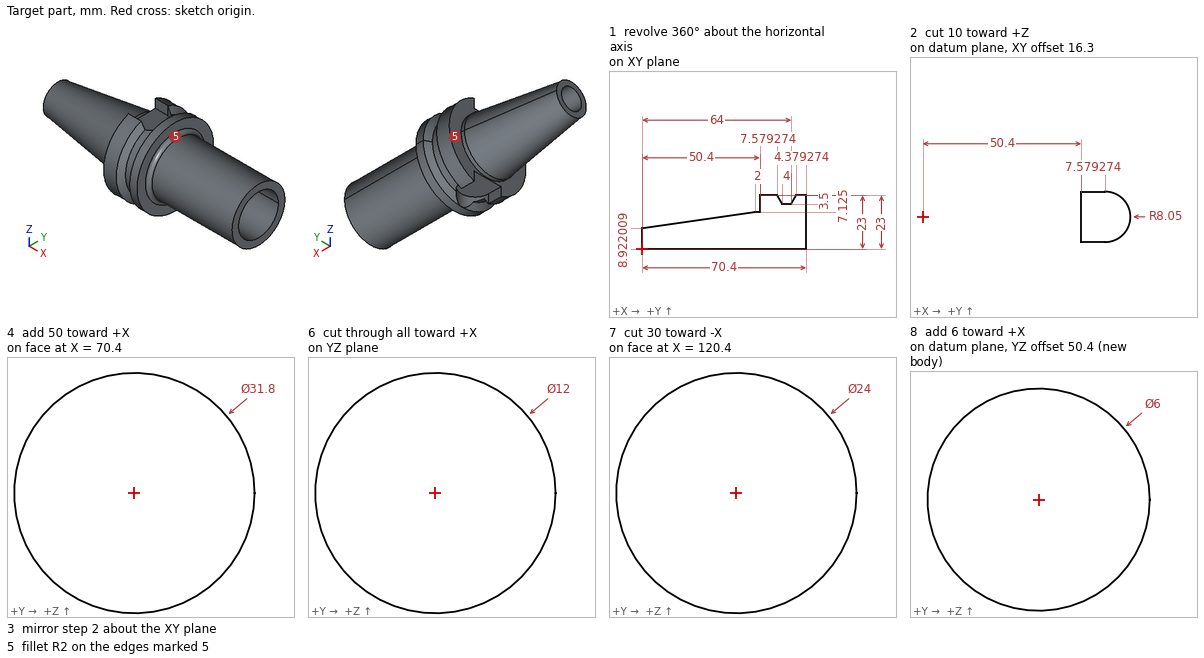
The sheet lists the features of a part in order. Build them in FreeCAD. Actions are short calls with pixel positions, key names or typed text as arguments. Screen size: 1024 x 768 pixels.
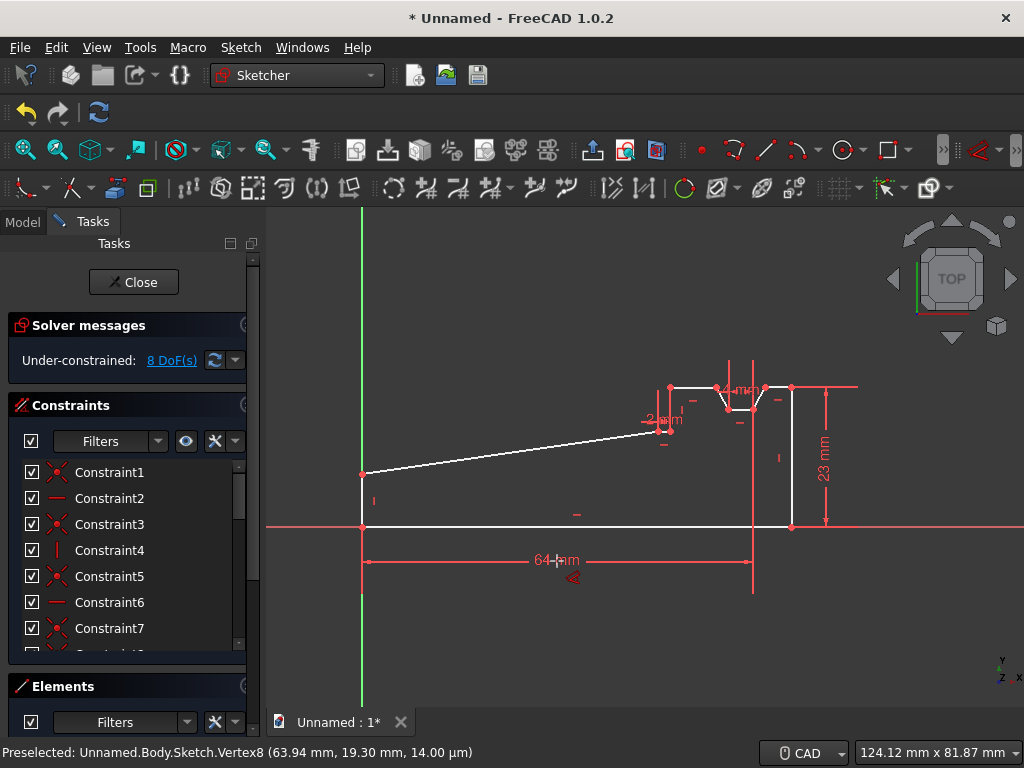
click(716, 388)
click(328, 458)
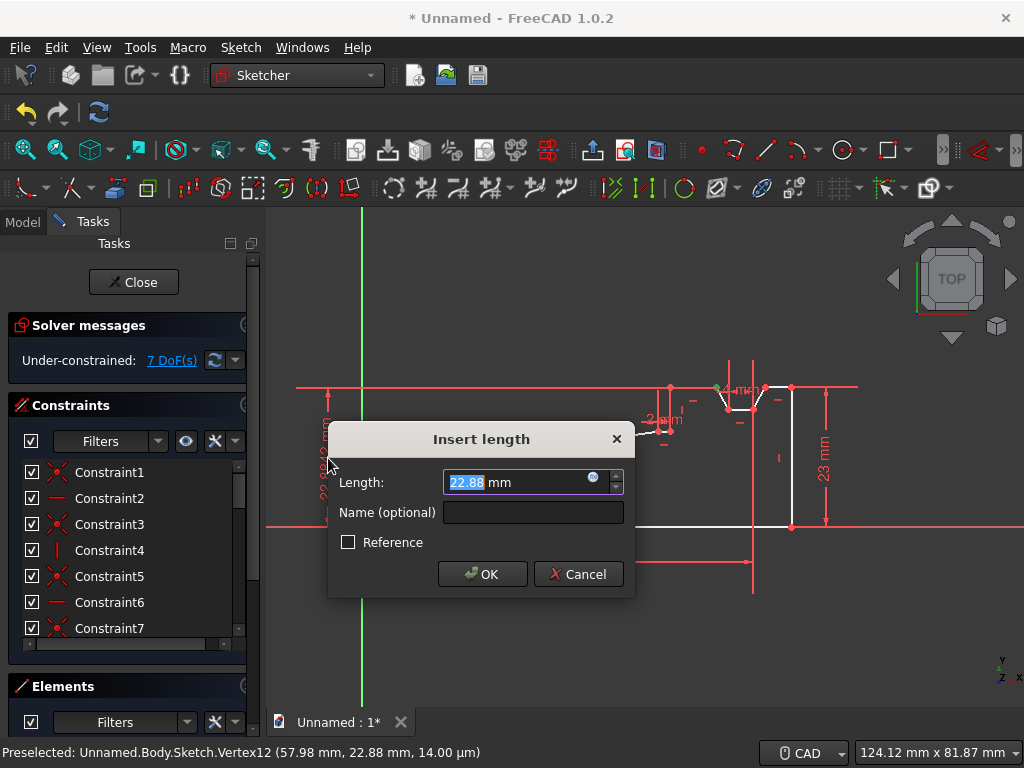
text(23)
key(Return)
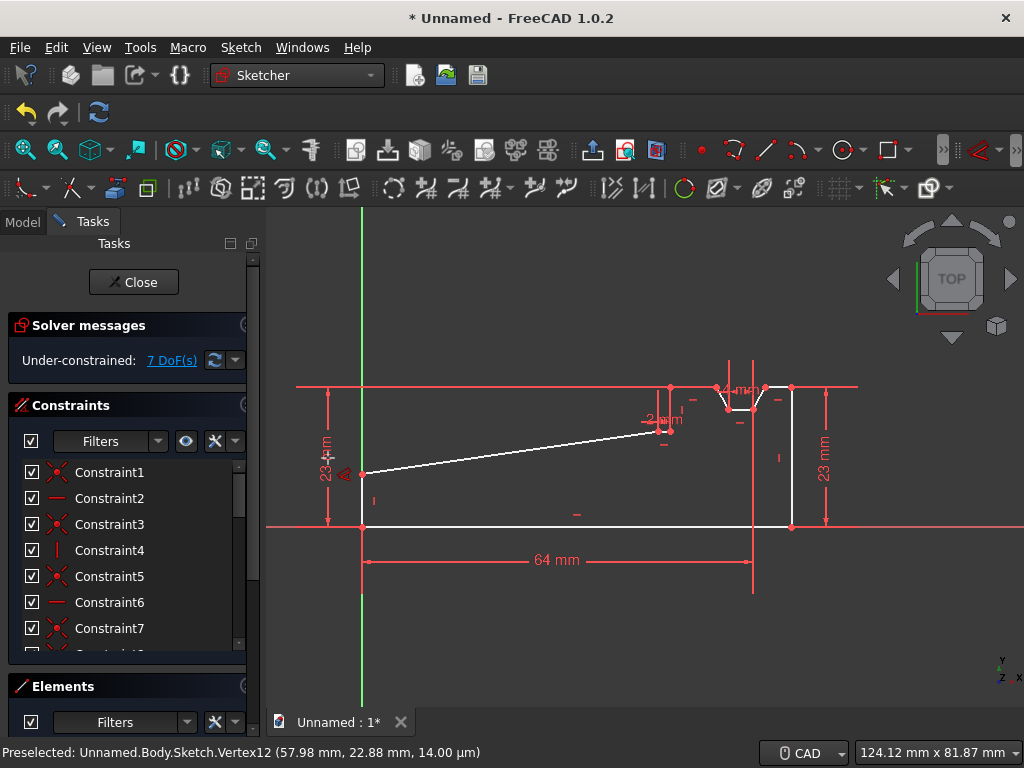
click(491, 527)
click(478, 561)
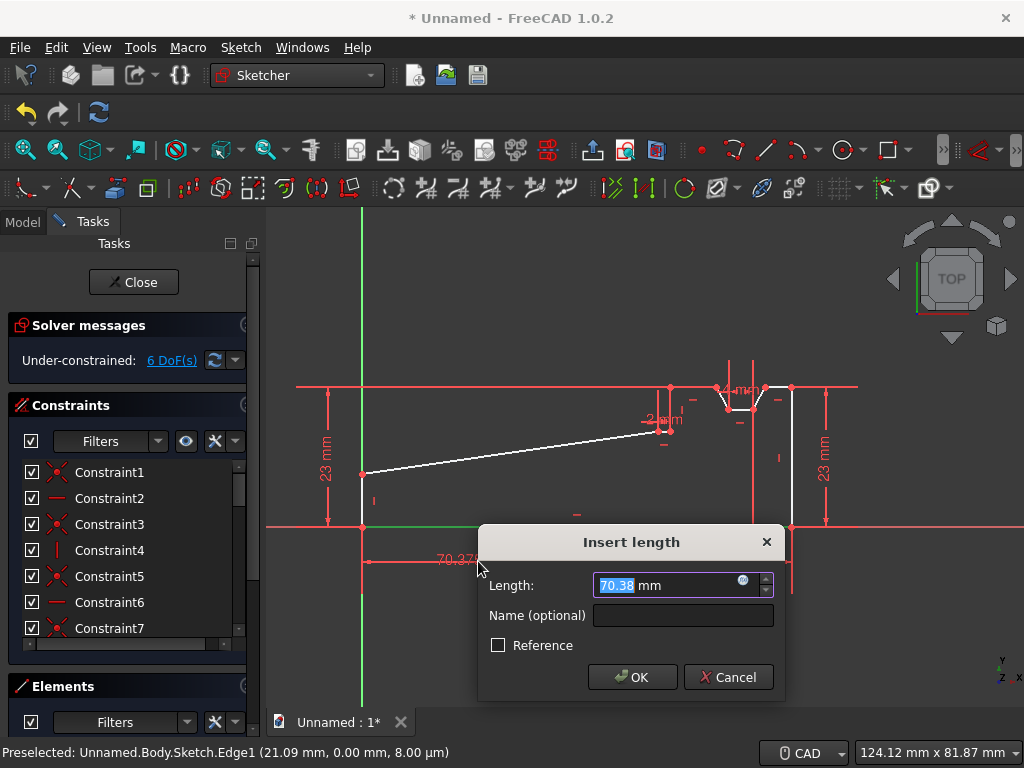
text(70.4)
key(Return)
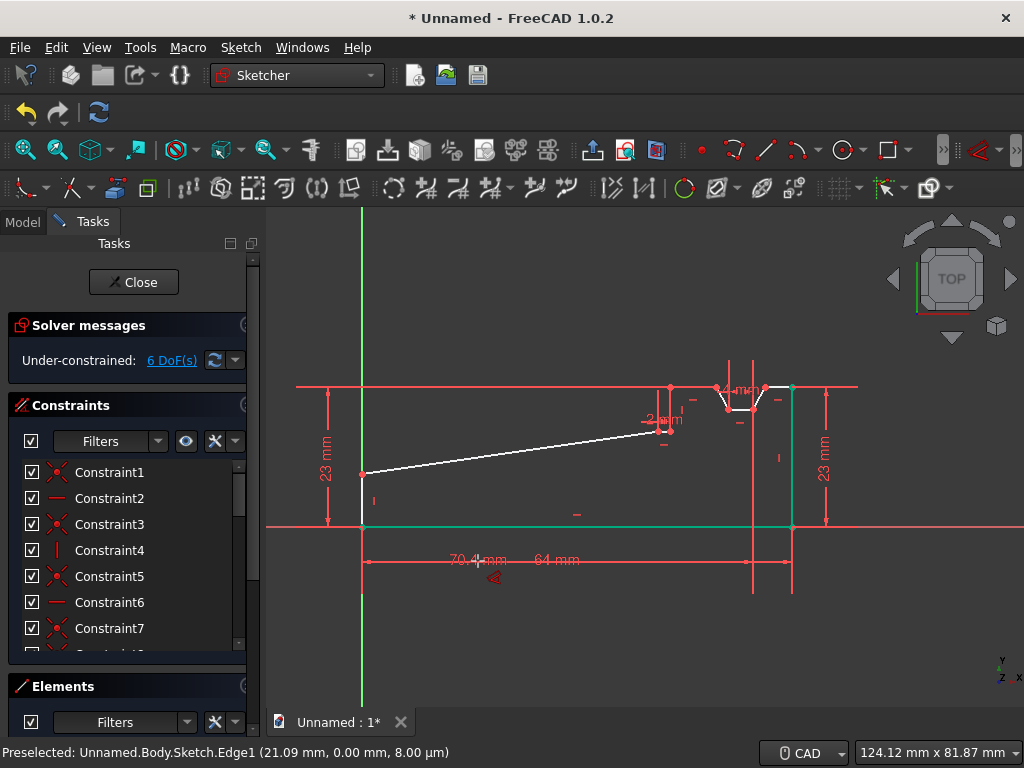
scroll(760, 396, up, 4)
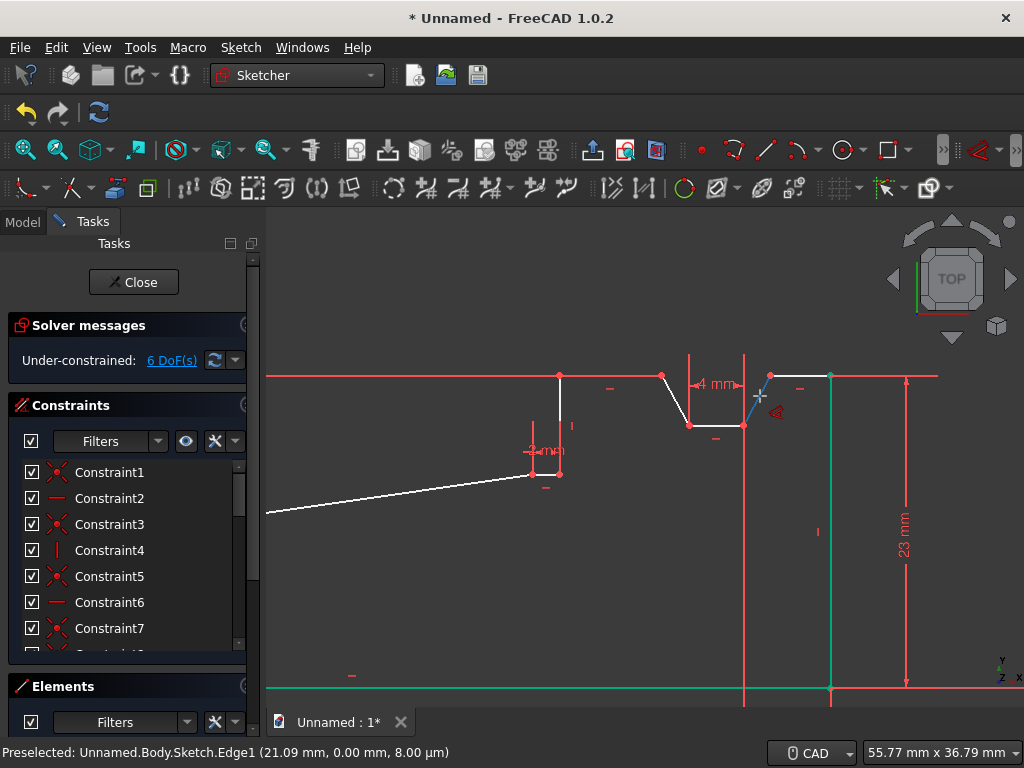
click(760, 396)
click(804, 401)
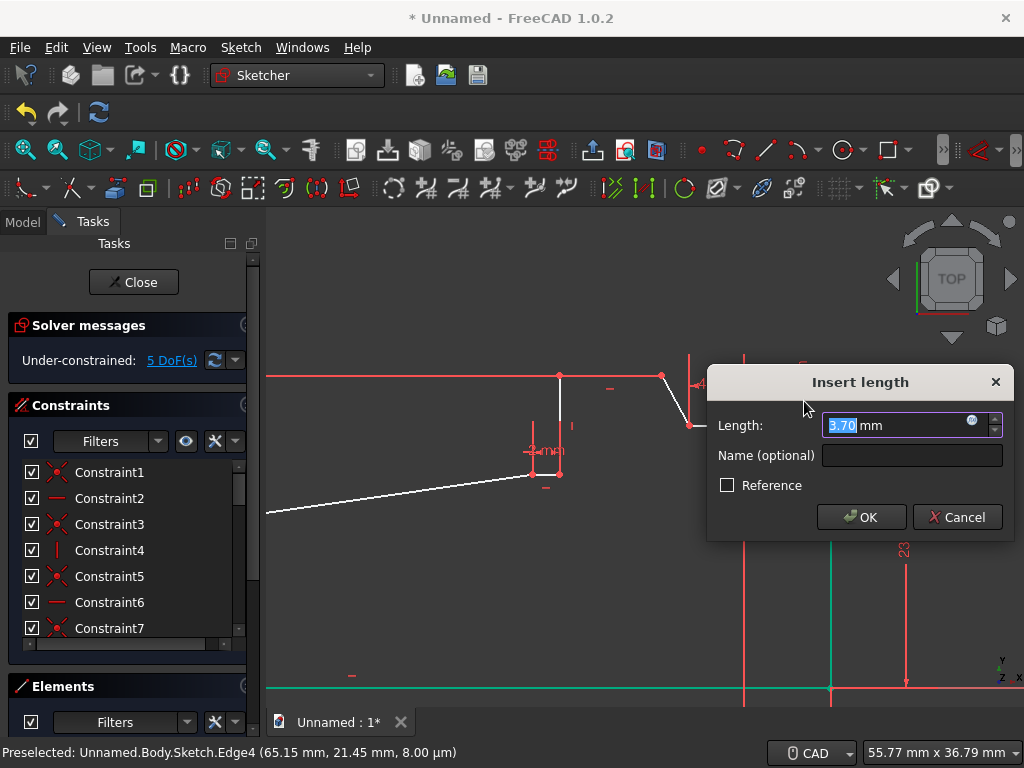
text(3.5)
key(Return)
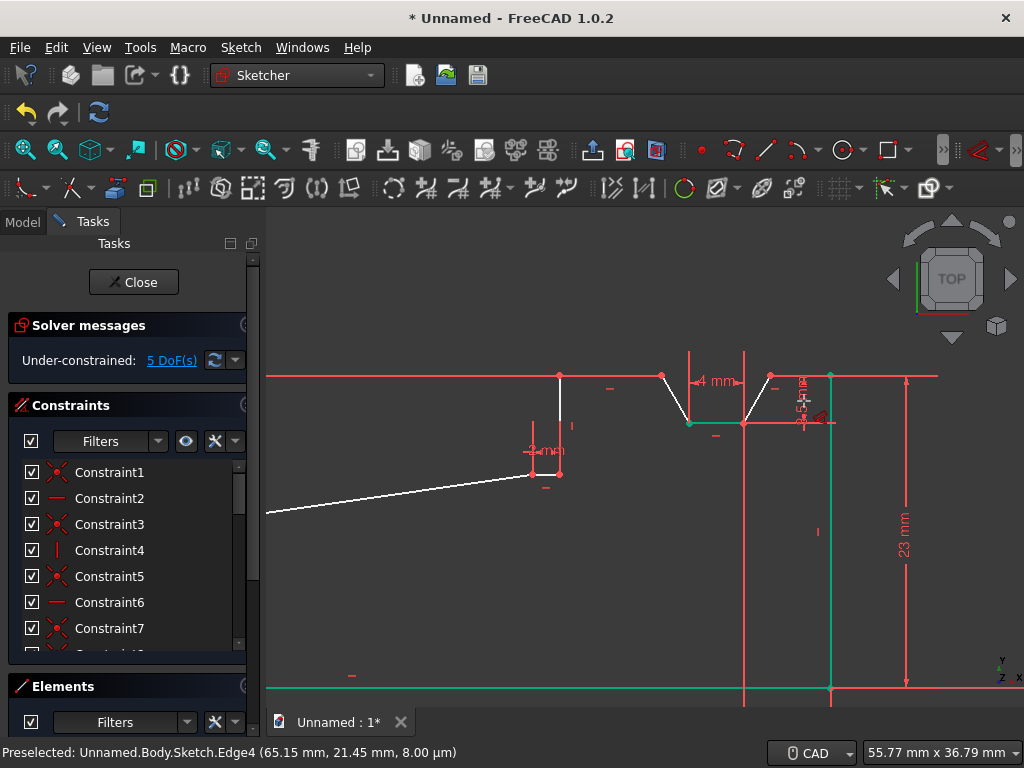
click(560, 405)
click(594, 425)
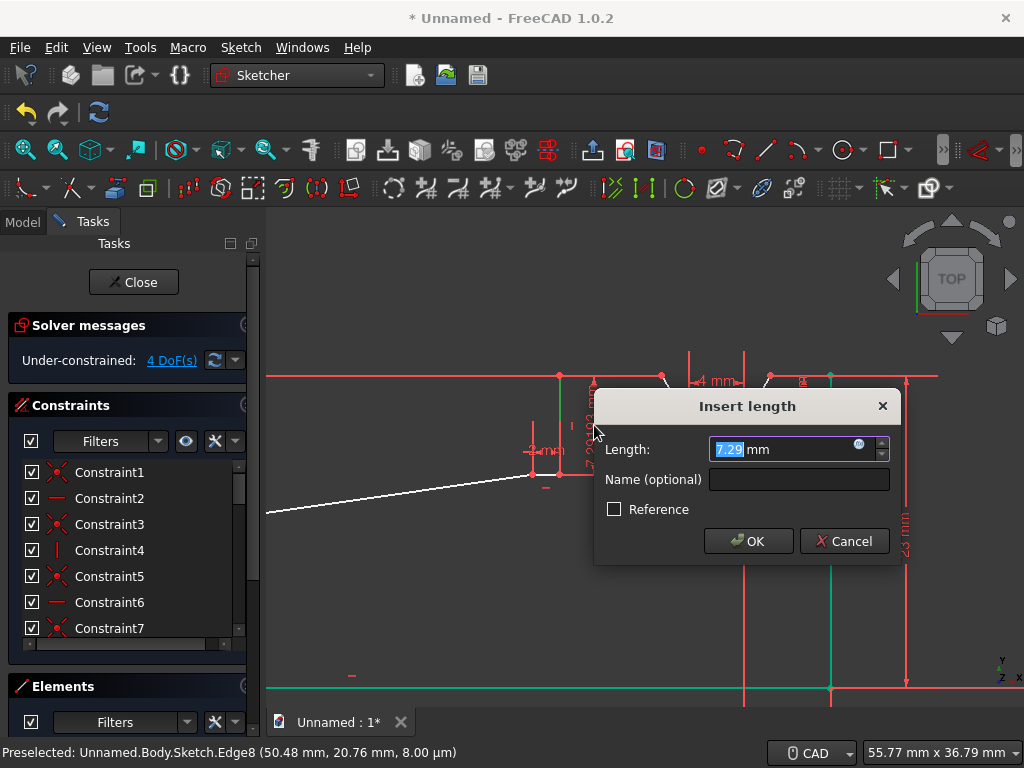
text(7.125)
key(Return)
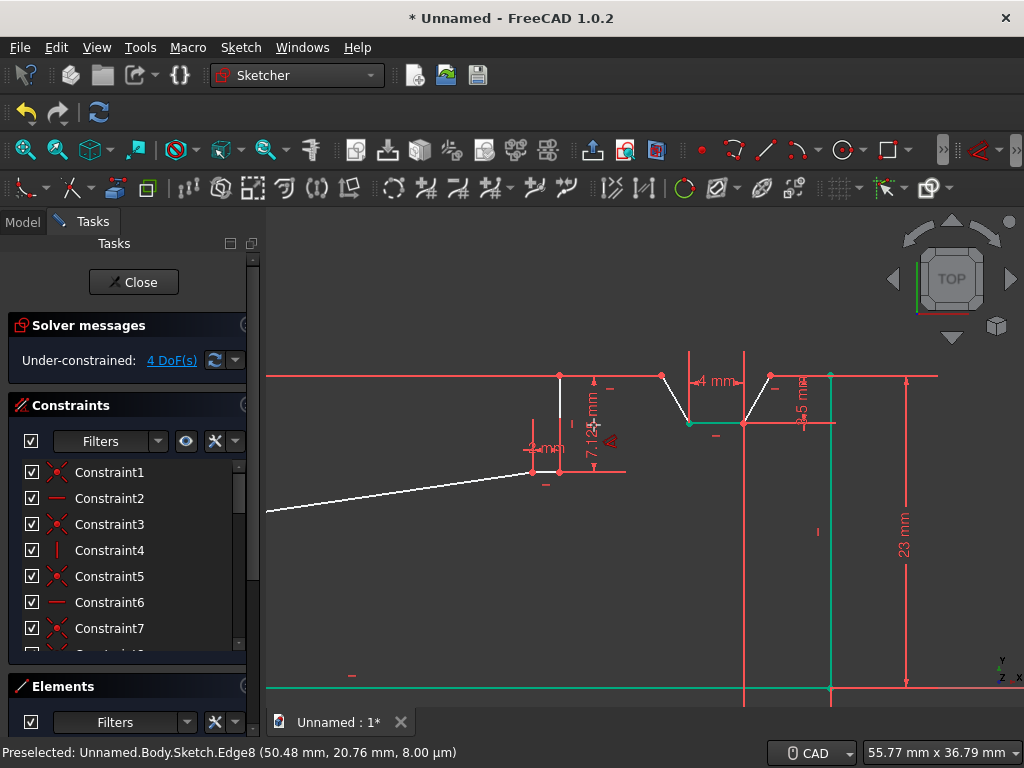
click(560, 376)
click(427, 342)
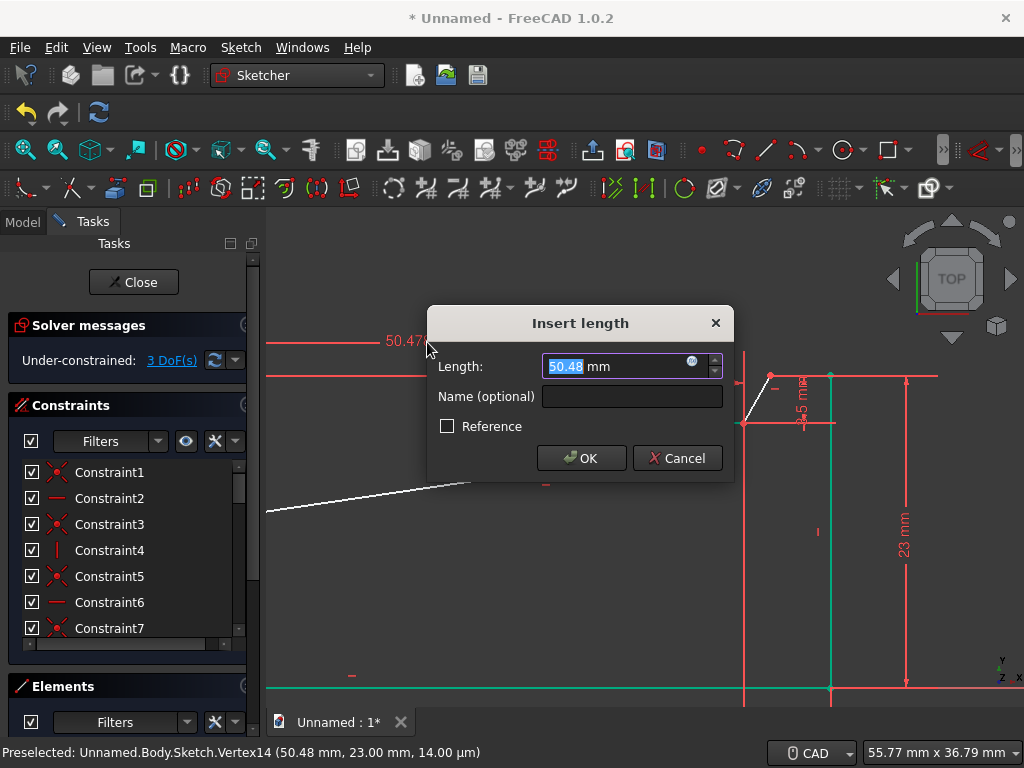
text(50.4)
key(Return)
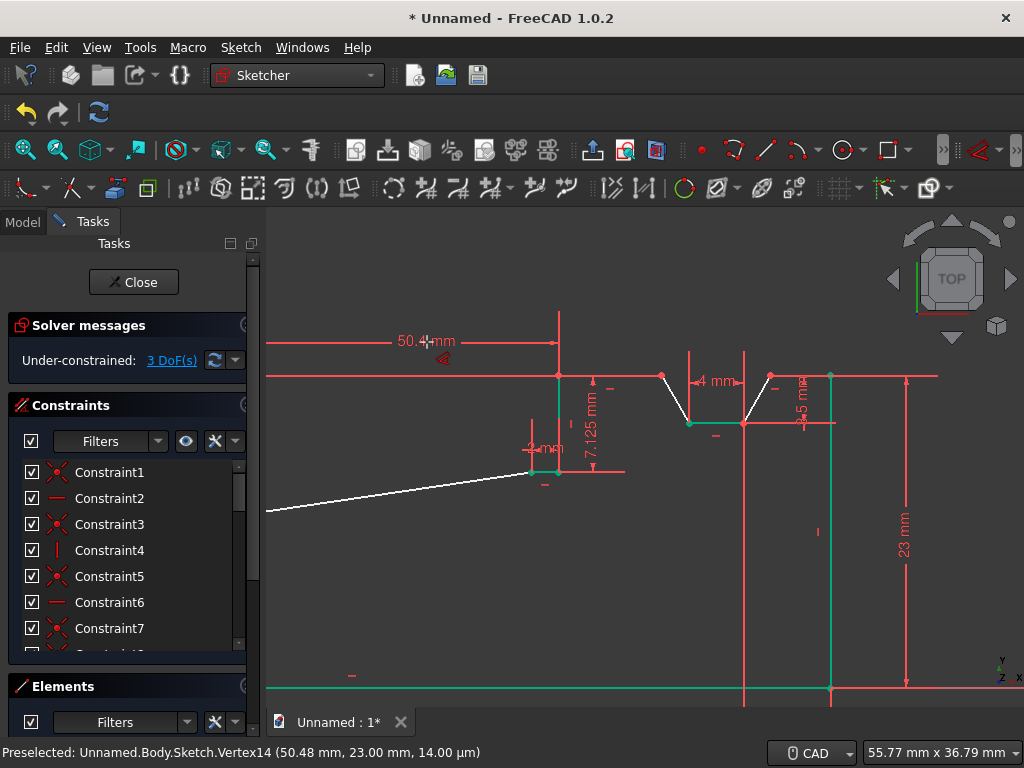
click(813, 376)
click(801, 342)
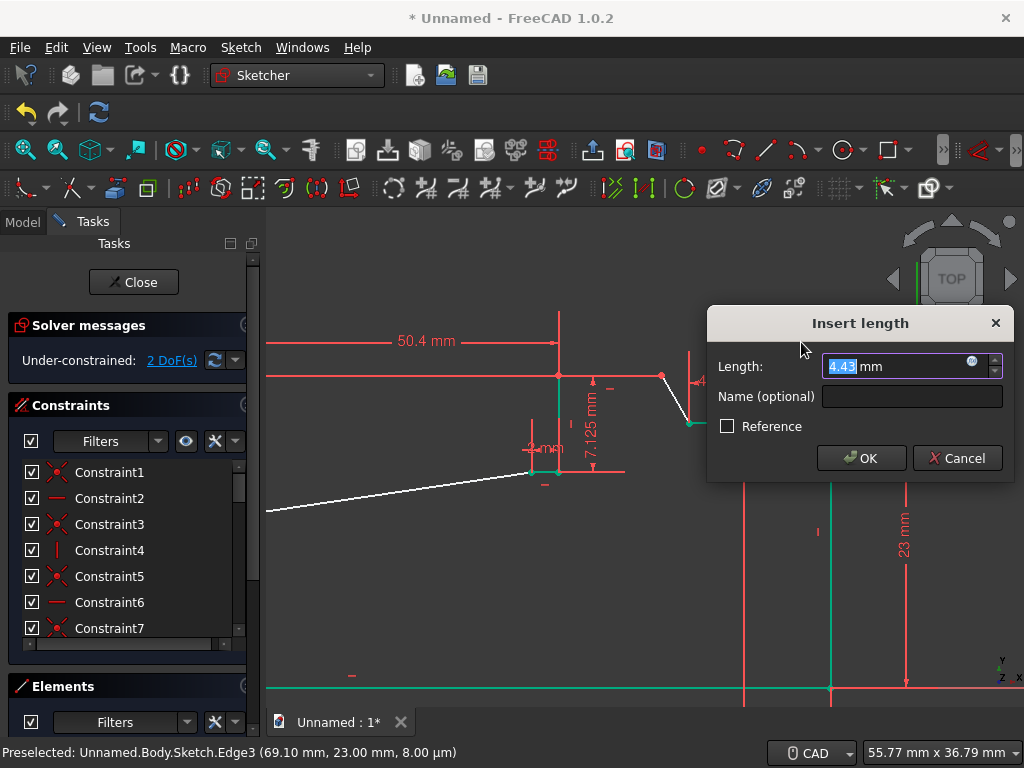
text(4.379274)
key(Return)